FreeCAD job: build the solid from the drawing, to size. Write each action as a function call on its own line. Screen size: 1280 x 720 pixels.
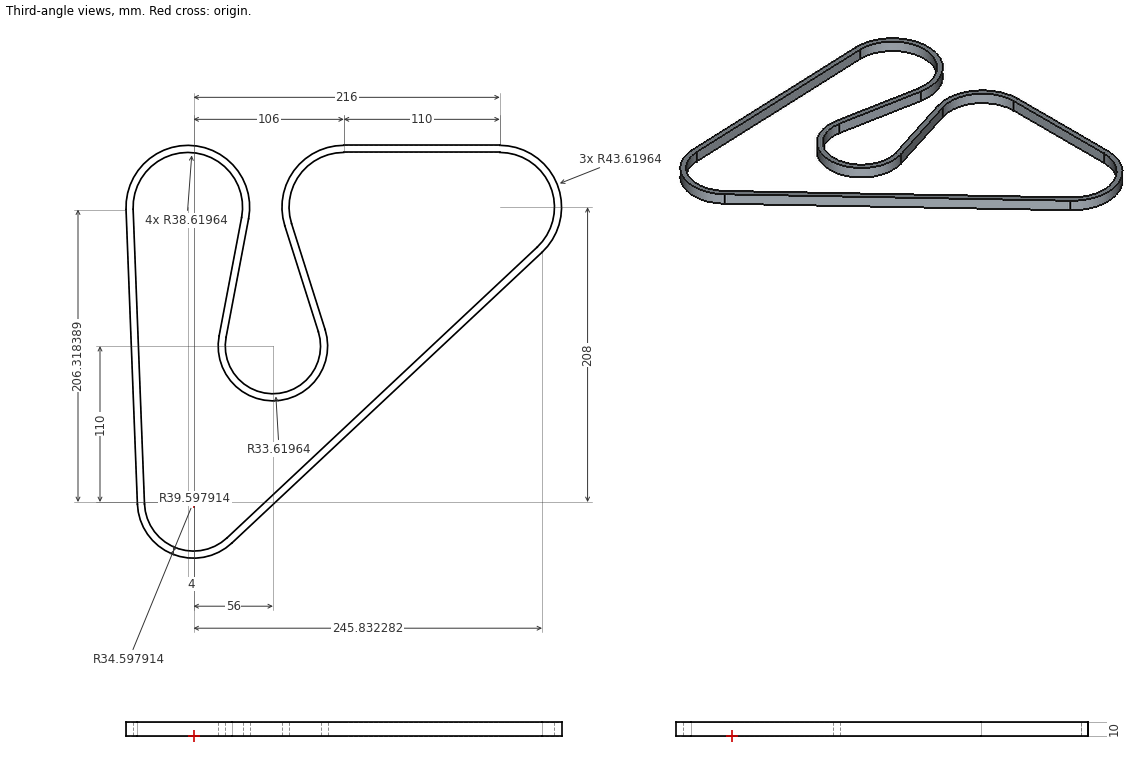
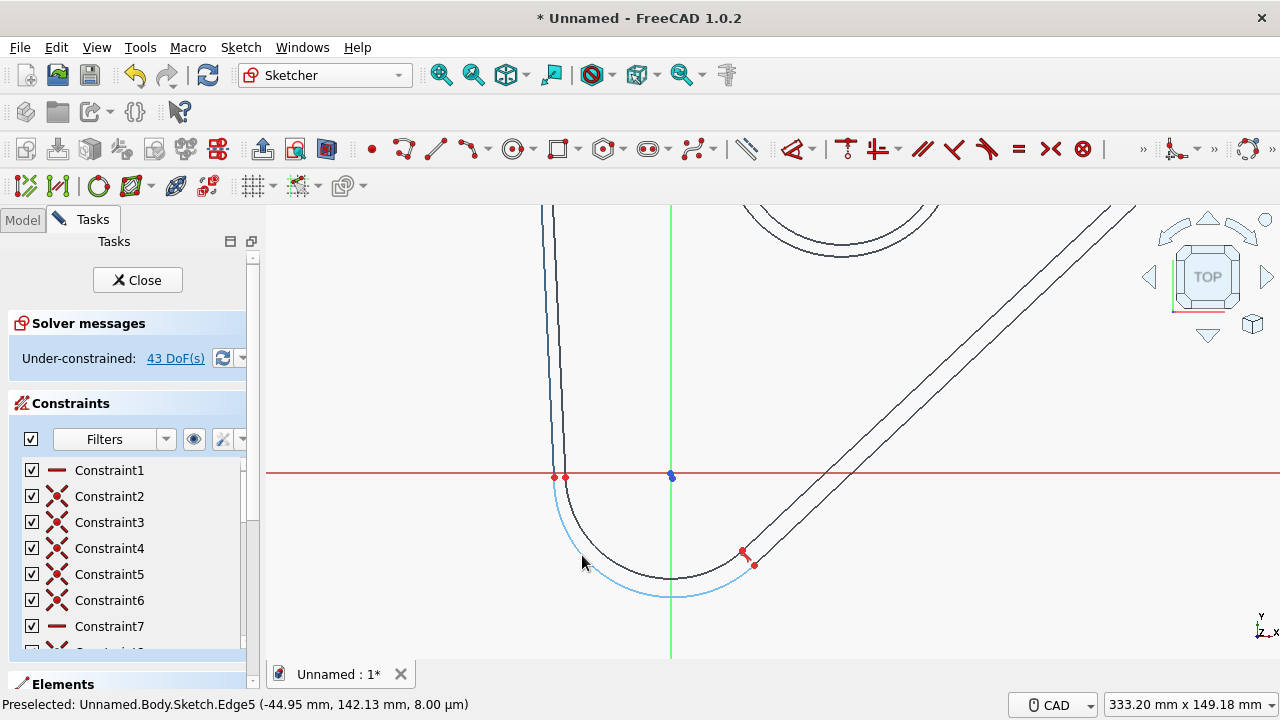
click(582, 555)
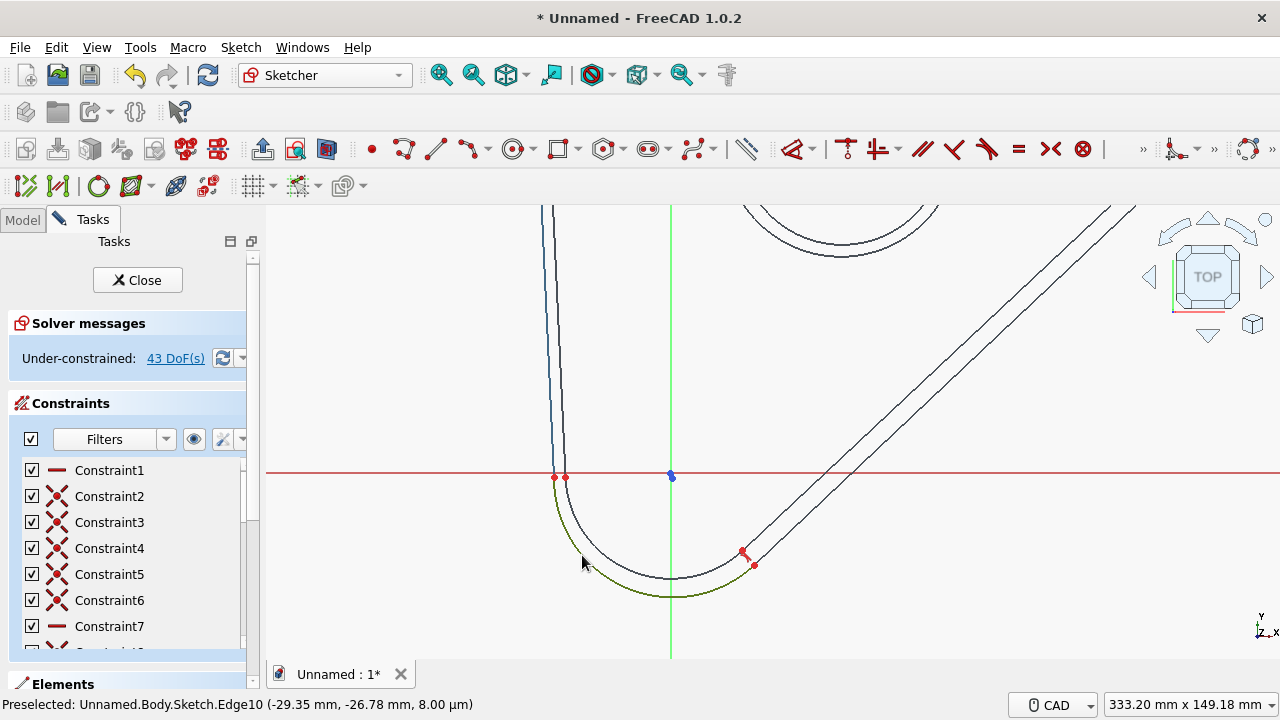
key(t)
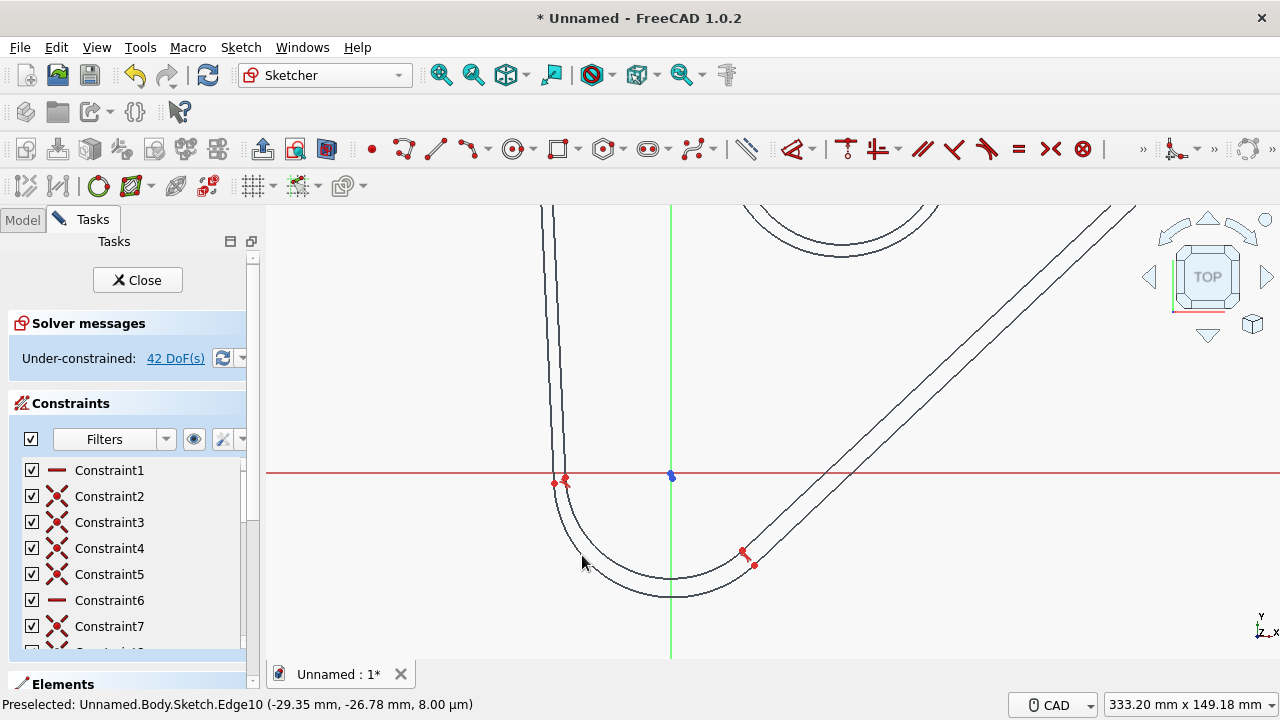
click(943, 363)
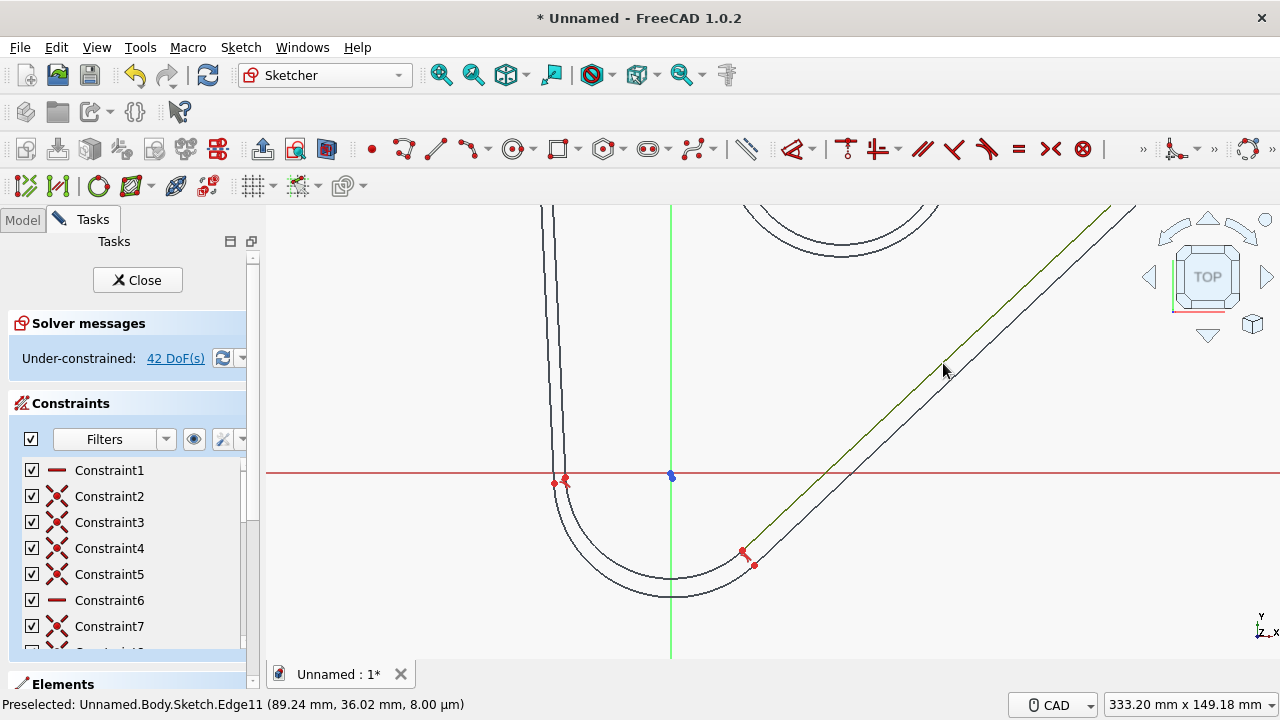
click(592, 543)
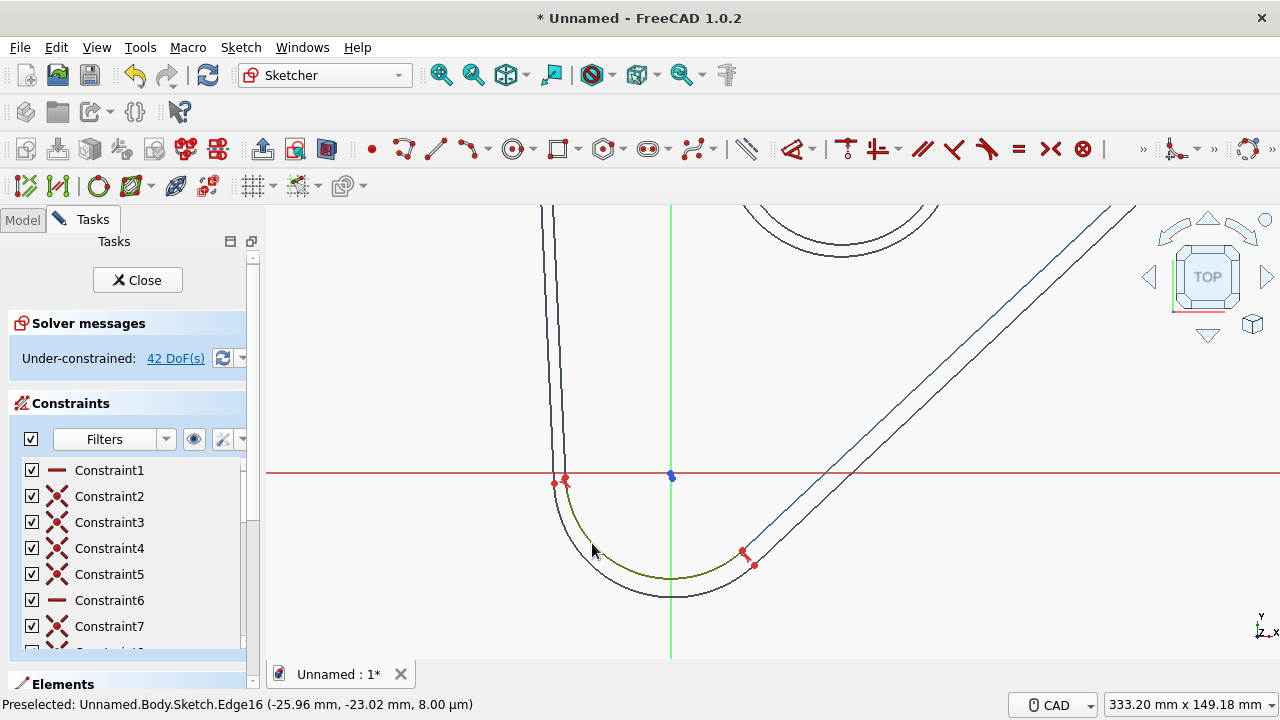
click(988, 150)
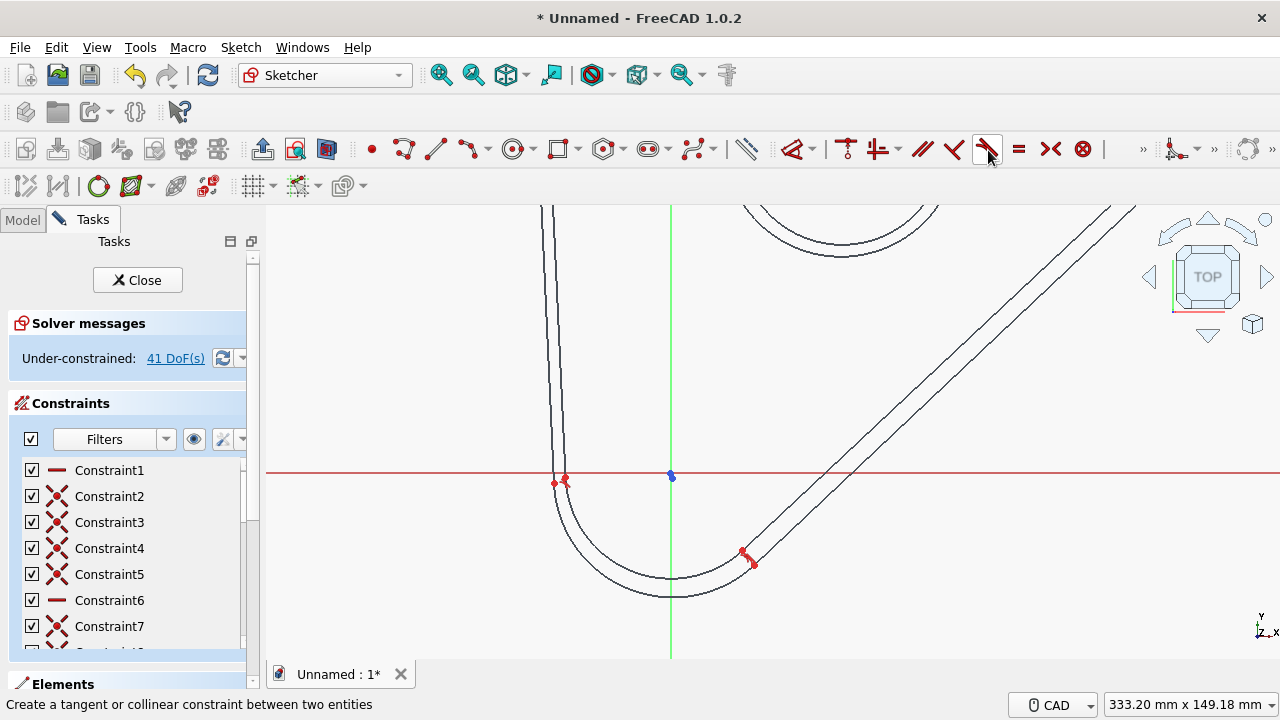
click(943, 363)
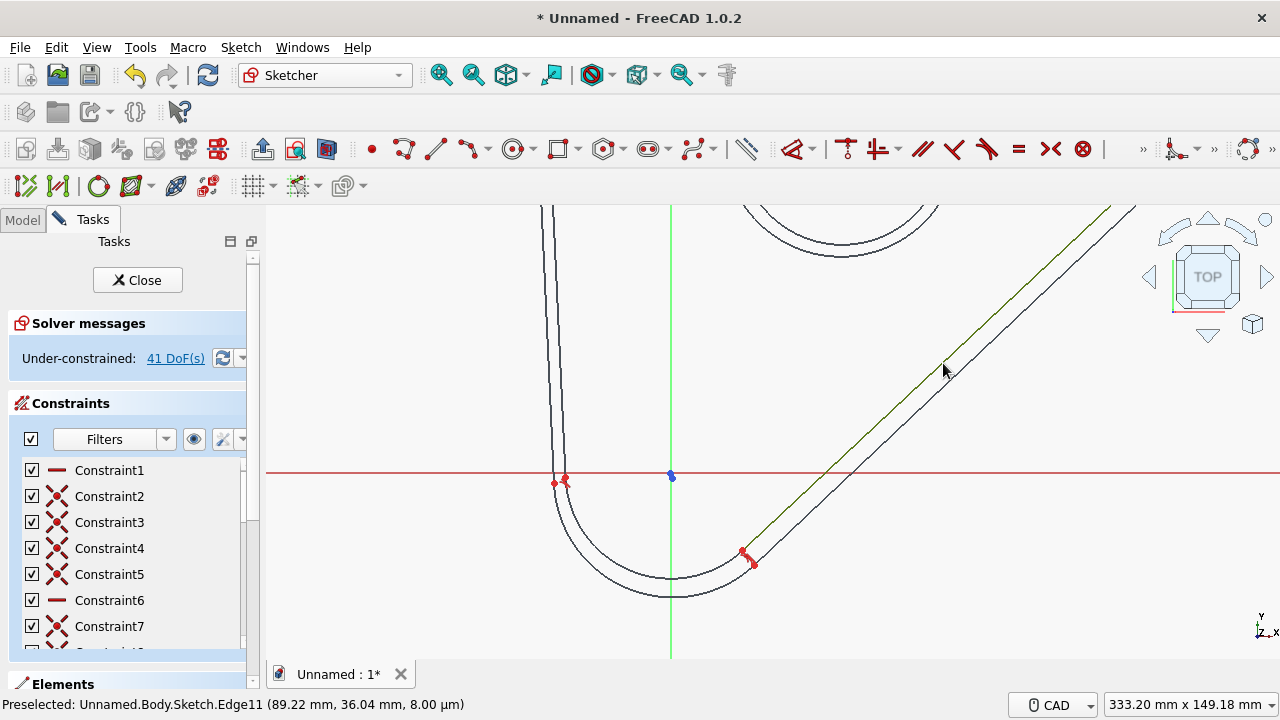
scroll(582, 555, down, 6)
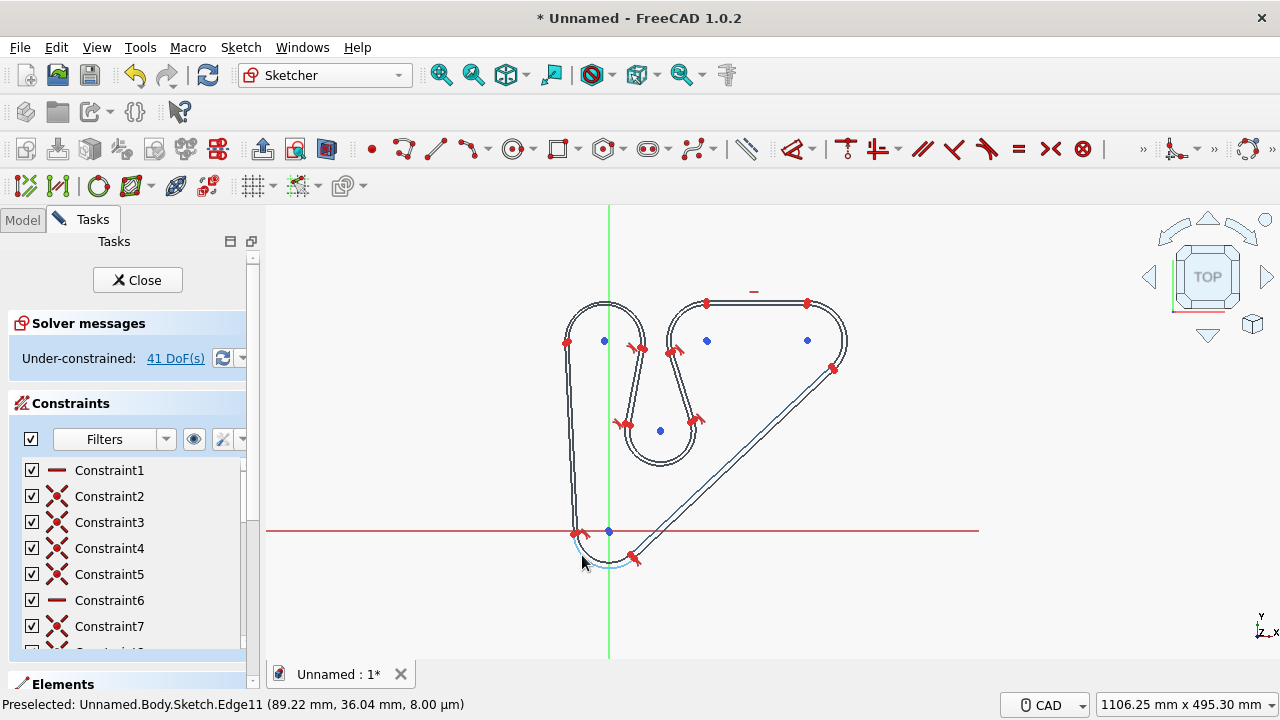
scroll(842, 344, up, 6)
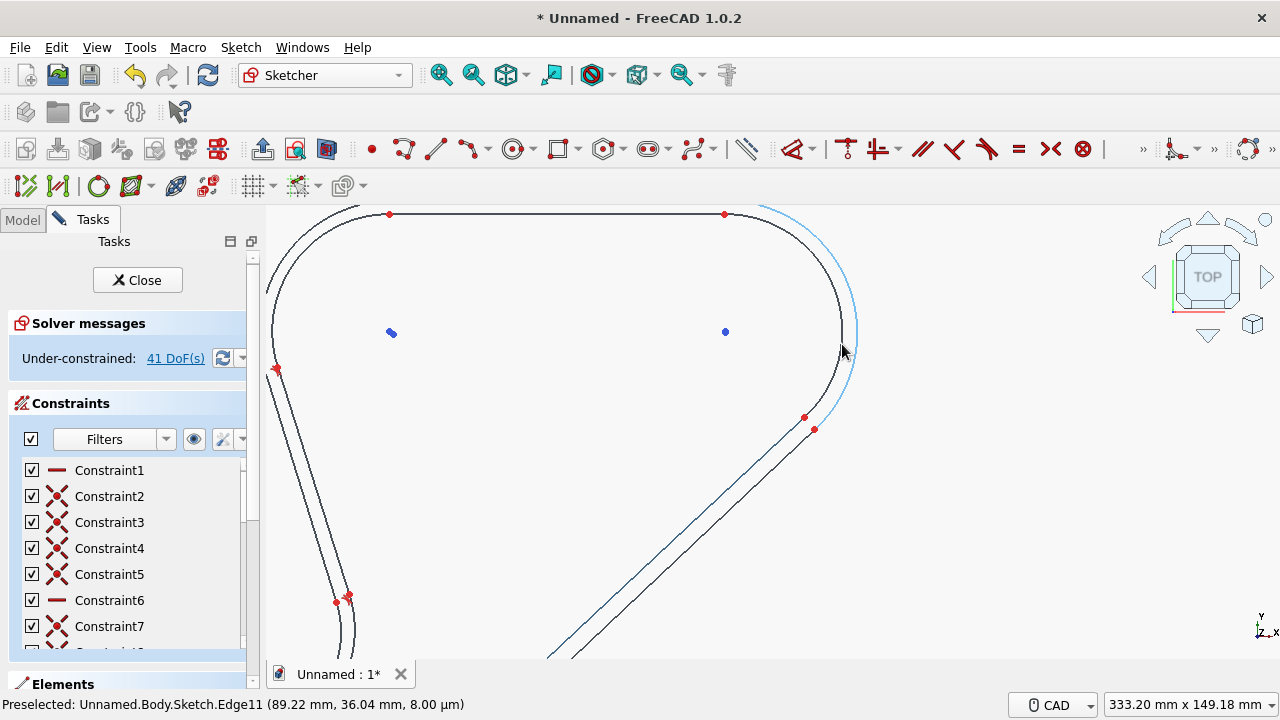
click(842, 344)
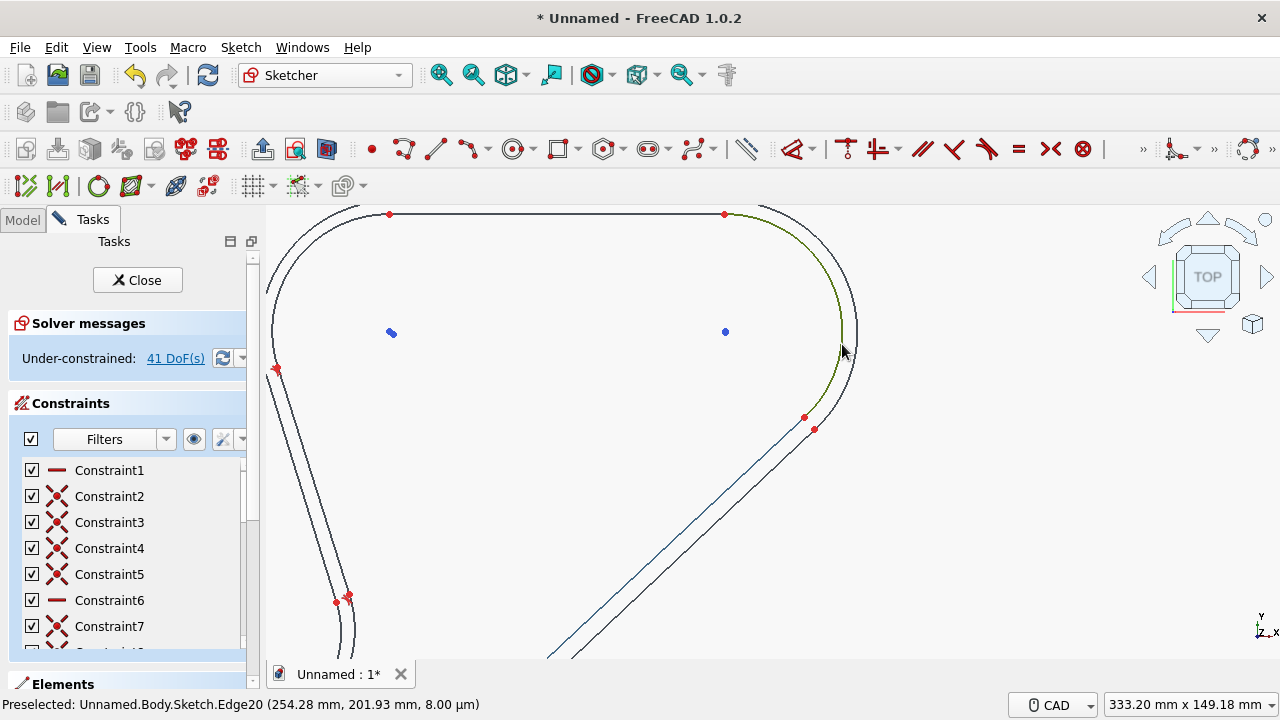
click(988, 150)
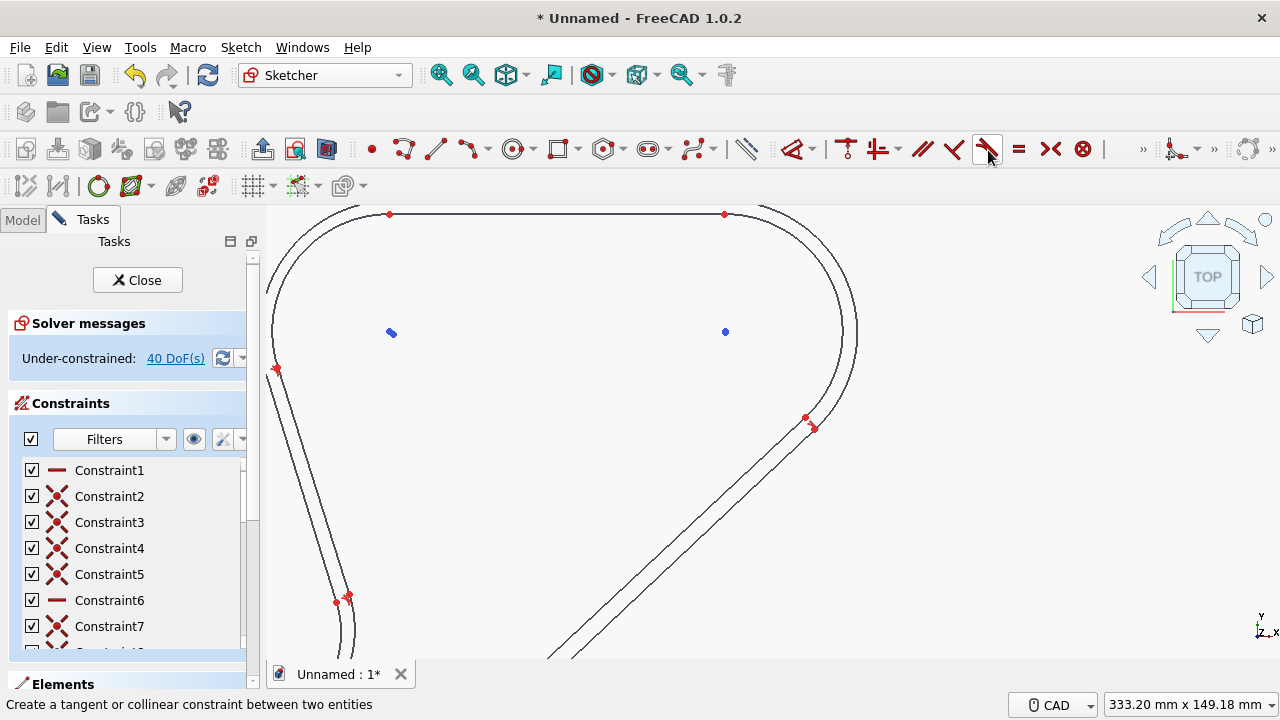
scroll(842, 344, down, 6)